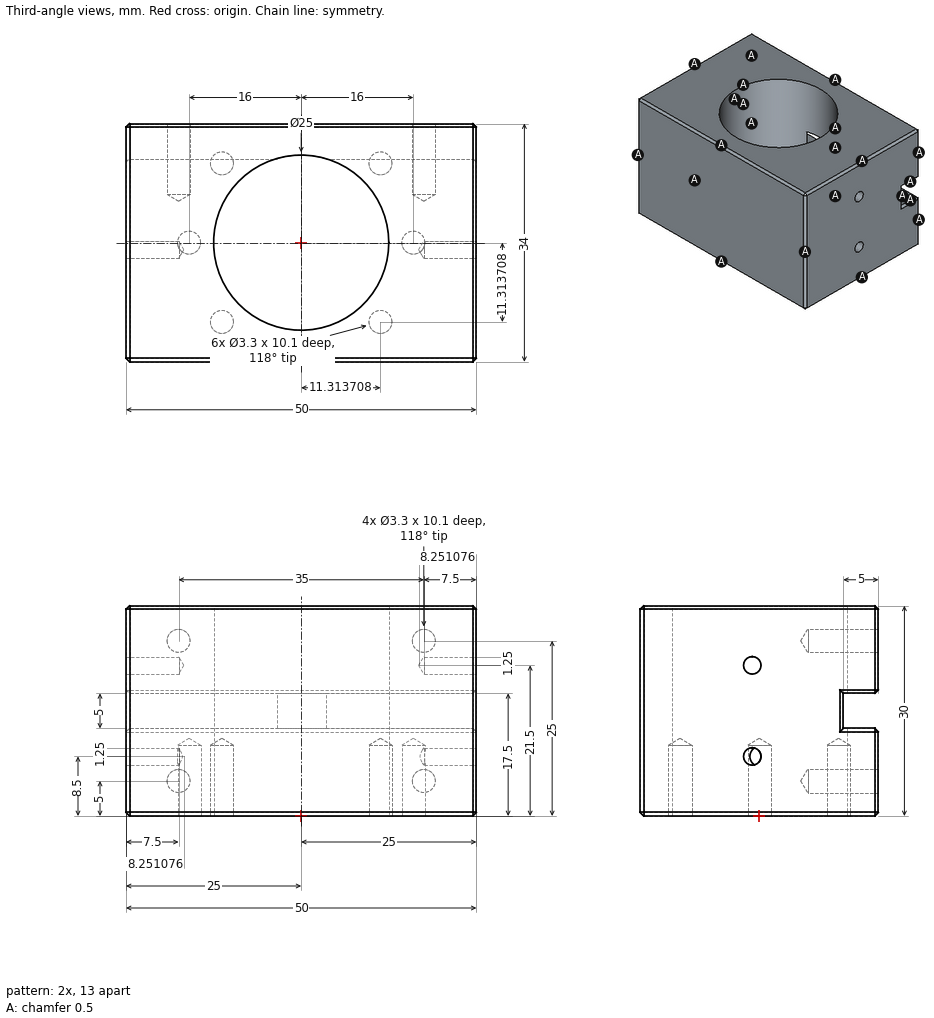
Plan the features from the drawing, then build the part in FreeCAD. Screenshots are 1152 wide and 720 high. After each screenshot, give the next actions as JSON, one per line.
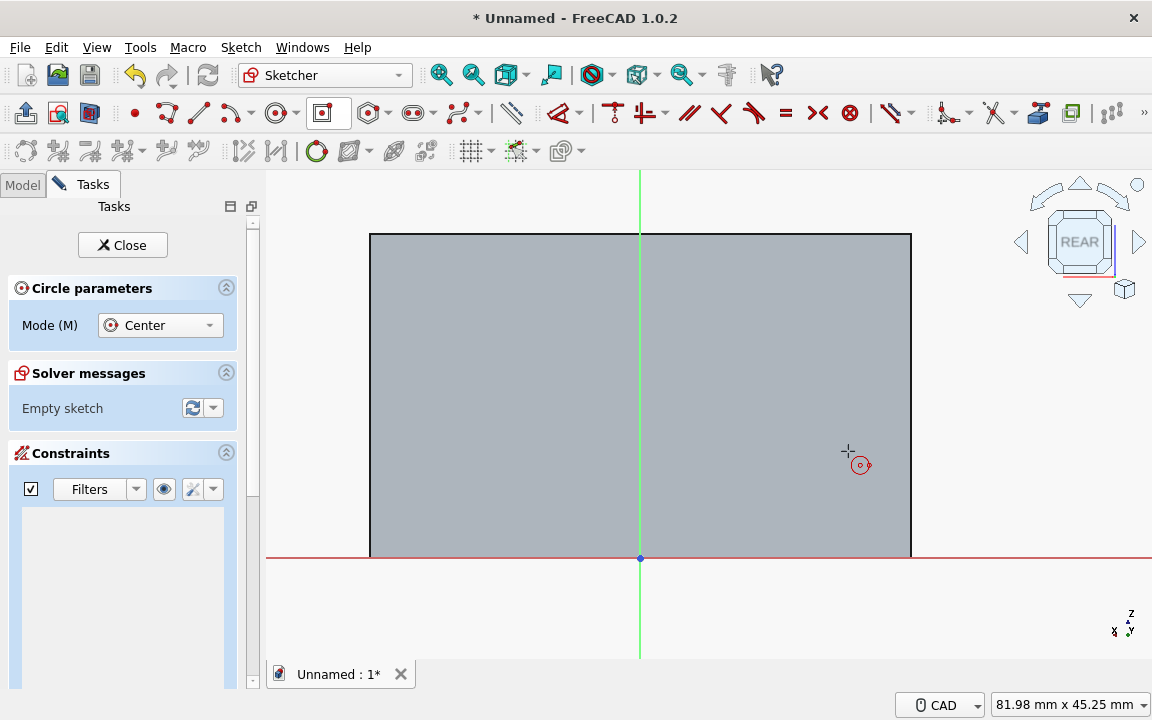
{"action": "scroll", "coordinate": [451, 288], "scroll_direction": "up", "scroll_amount": 2}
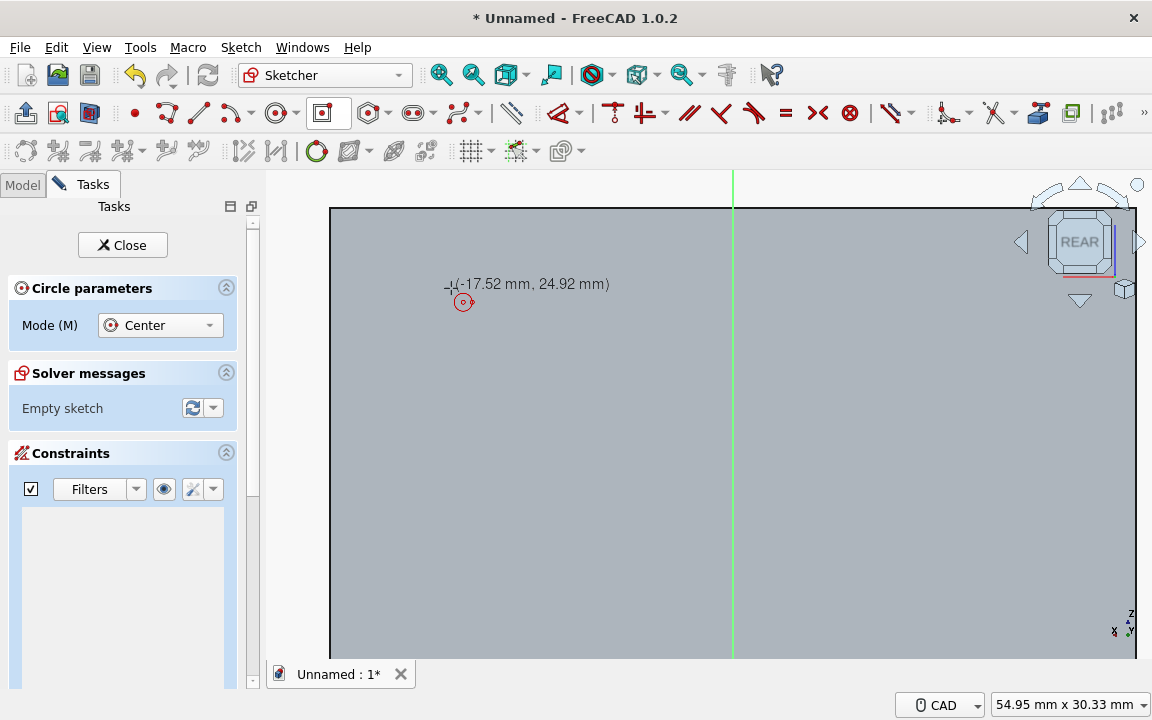
{"action": "left_click", "coordinate": [451, 288]}
{"action": "mouse_move", "coordinate": [470, 269]}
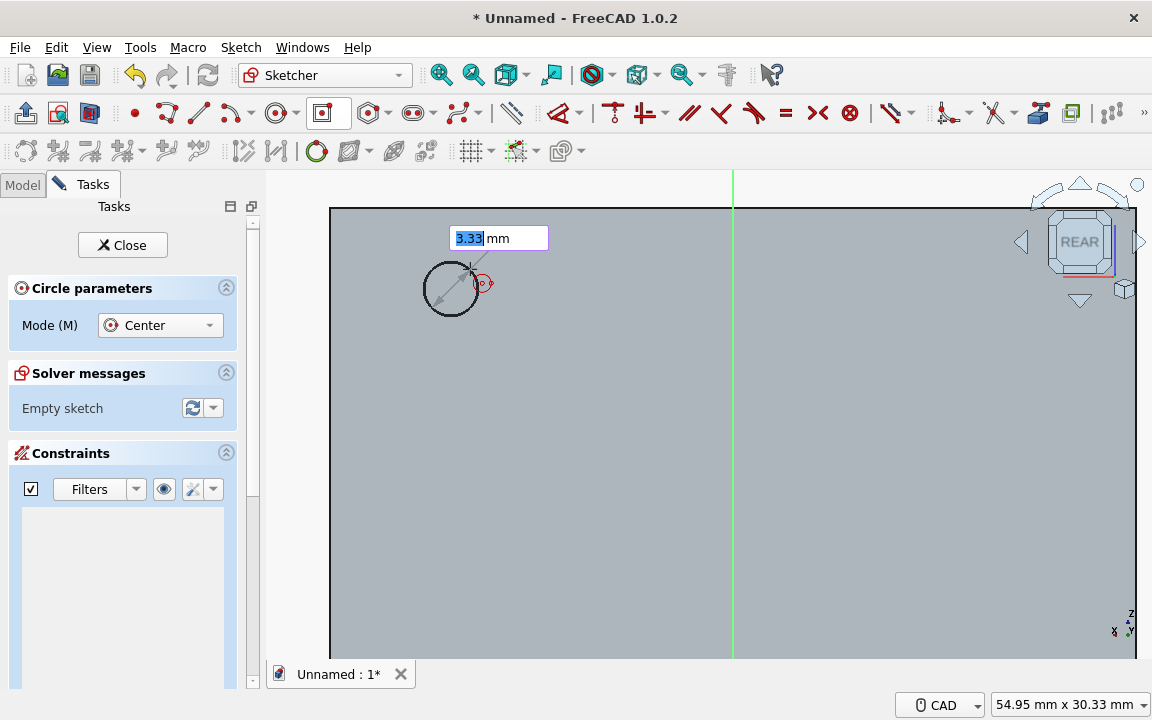
{"action": "type", "text": "3.3"}
{"action": "key", "text": "Return"}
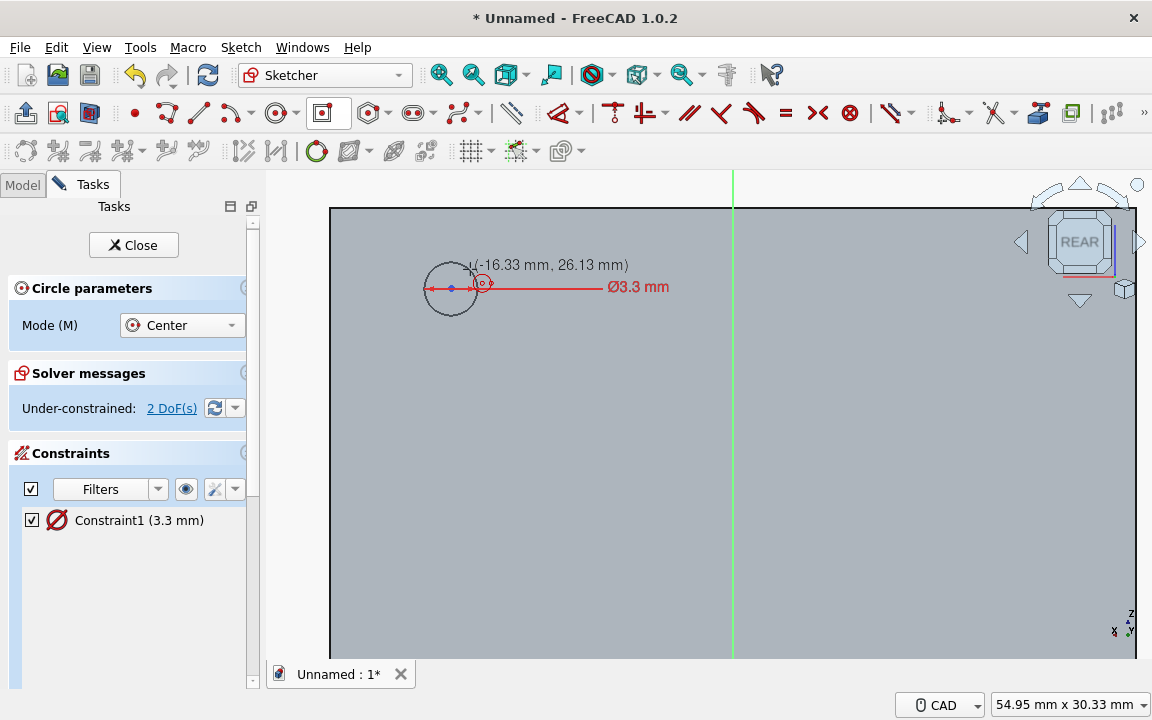
{"action": "scroll", "coordinate": [452, 289], "scroll_direction": "down", "scroll_amount": 2}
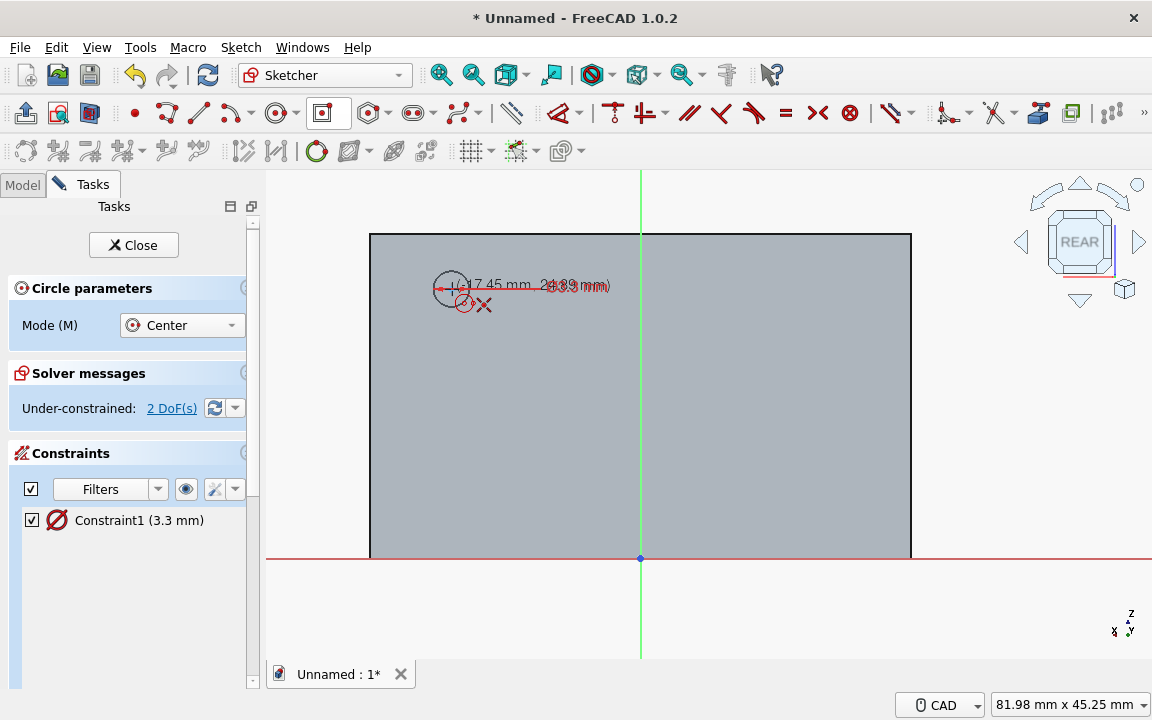
{"action": "scroll", "coordinate": [830, 289], "scroll_direction": "up", "scroll_amount": 2}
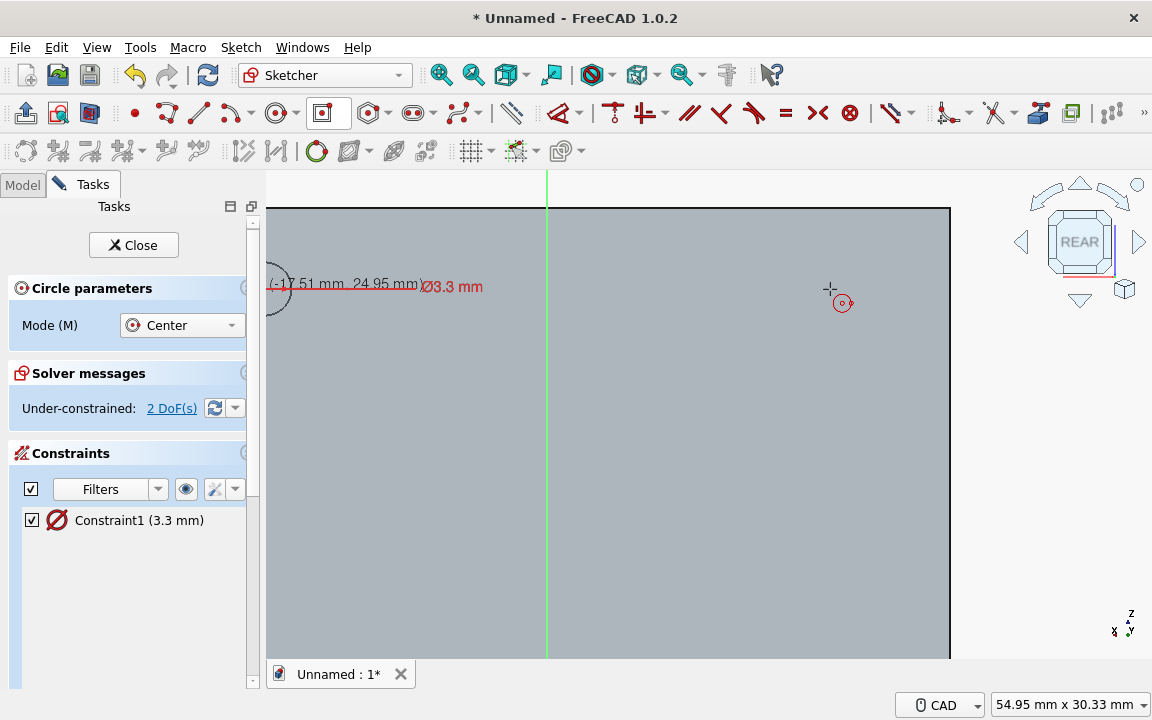
{"action": "left_click", "coordinate": [829, 288]}
{"action": "mouse_move", "coordinate": [848, 269]}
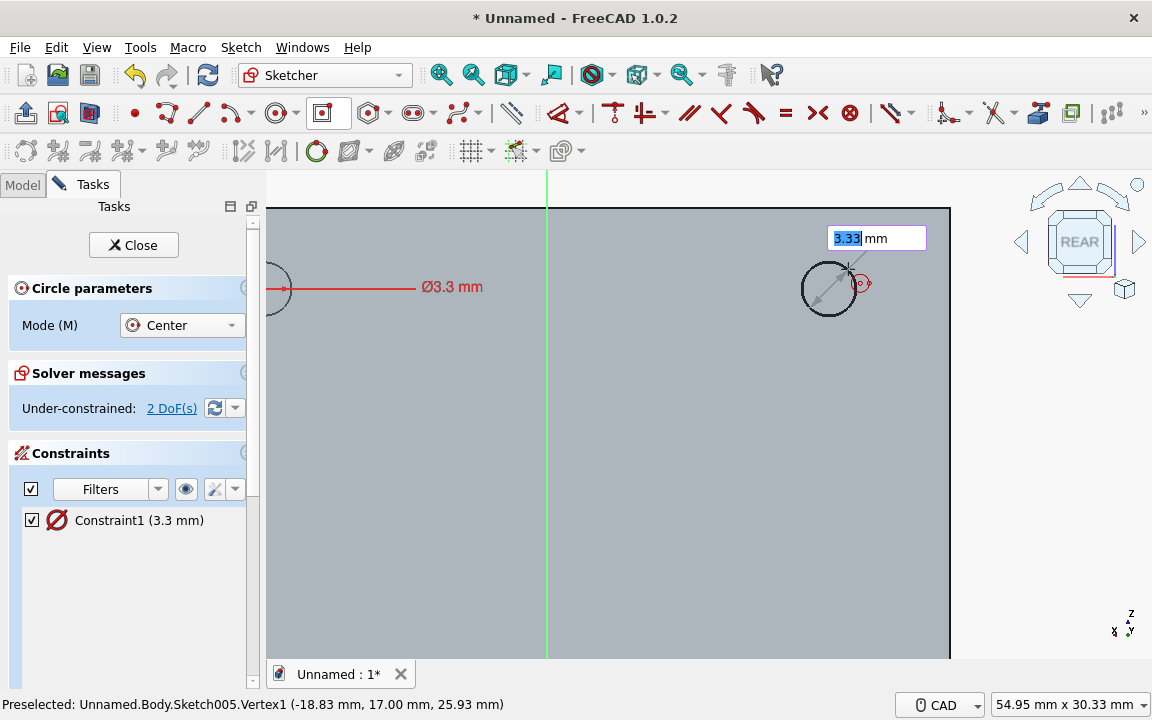
{"action": "type", "text": "3.3"}
{"action": "key", "text": "Return"}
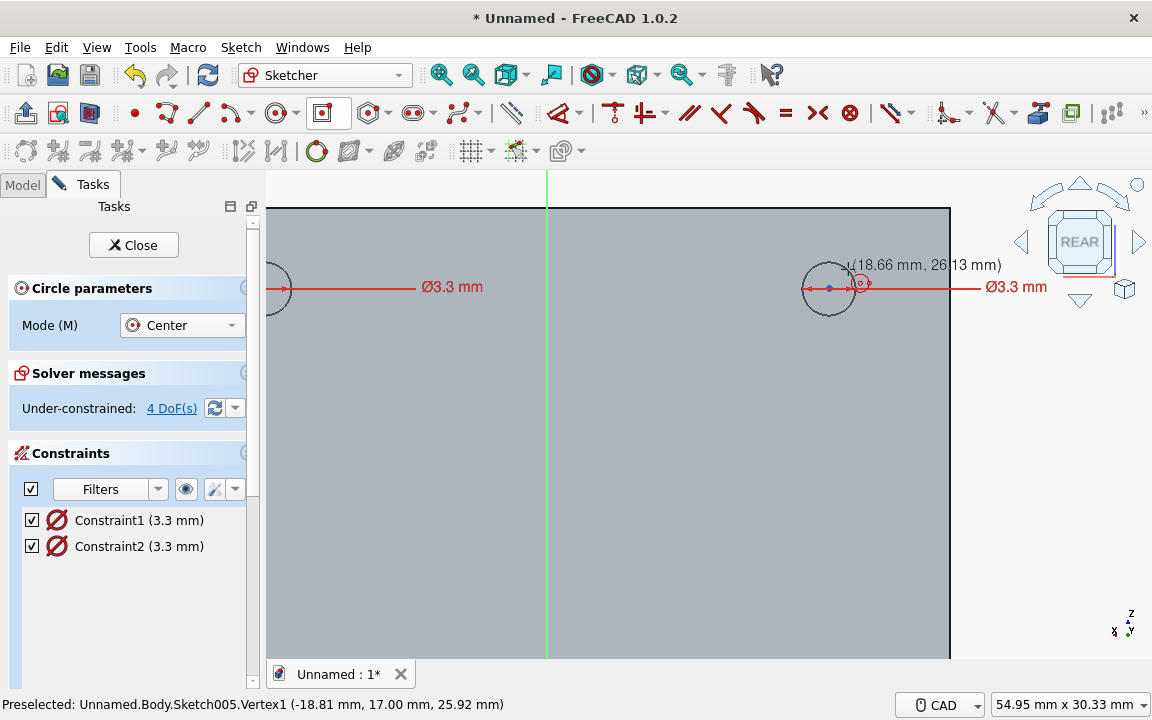
{"action": "left_click", "coordinate": [829, 611]}
{"action": "mouse_move", "coordinate": [848, 592]}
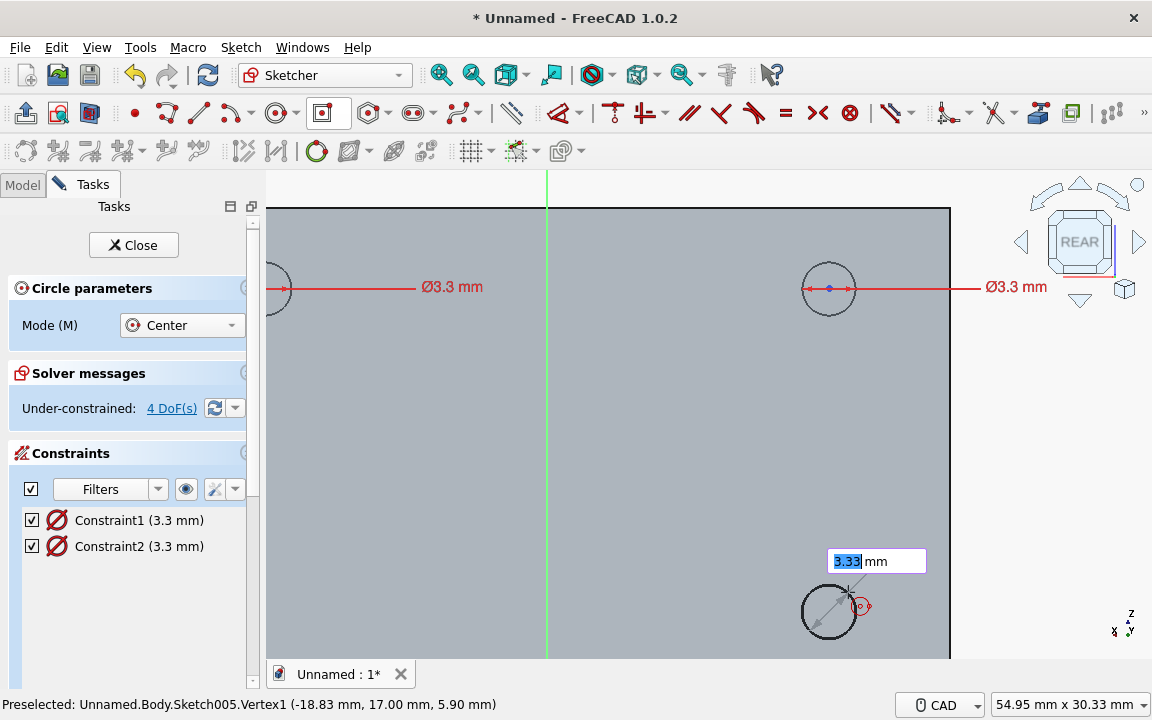
{"action": "type", "text": "3.3"}
{"action": "key", "text": "Return"}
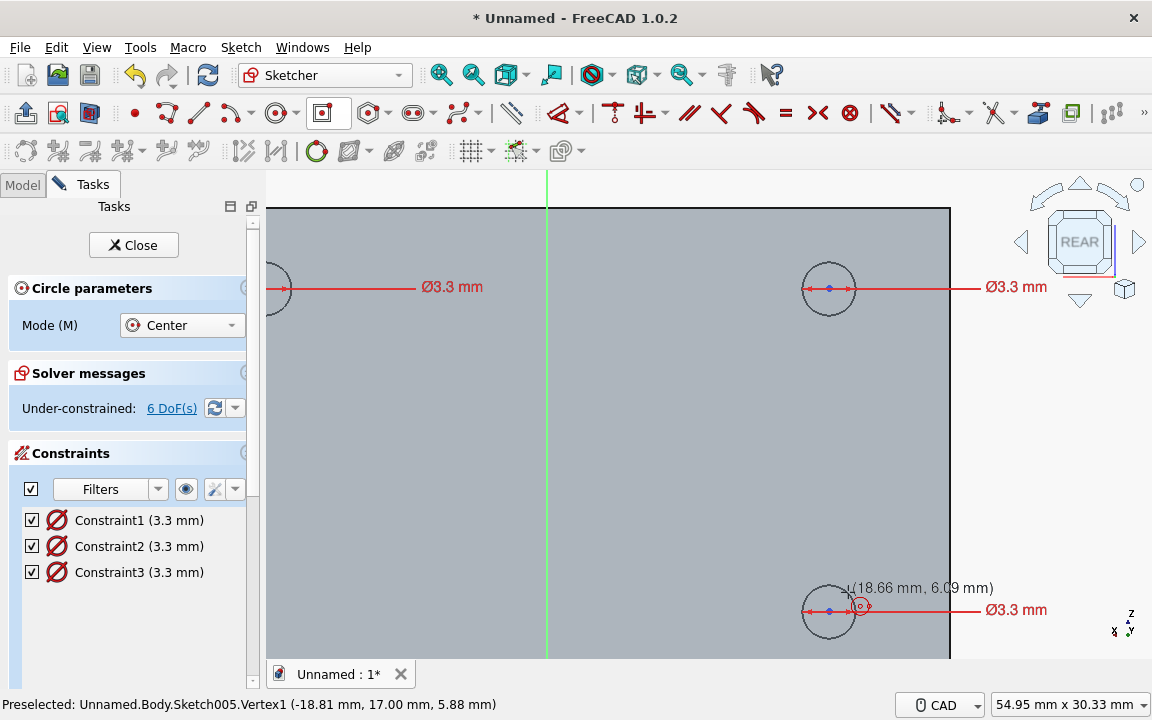
{"action": "scroll", "coordinate": [830, 289], "scroll_direction": "down", "scroll_amount": 2}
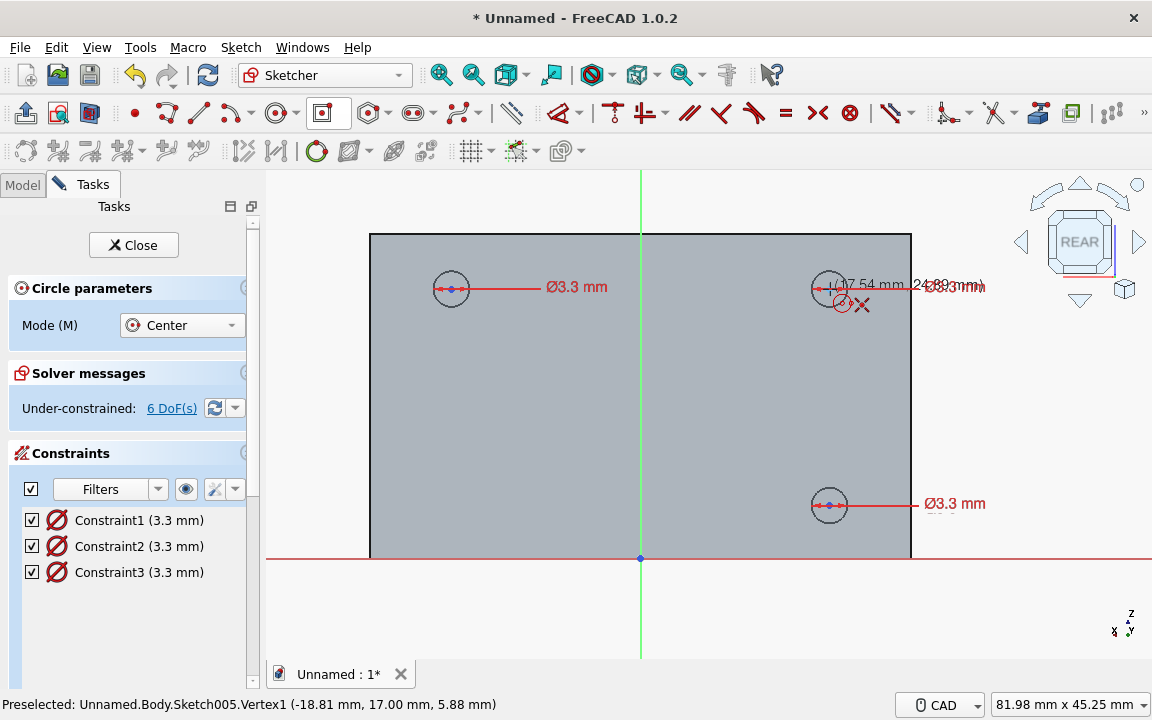
{"action": "scroll", "coordinate": [452, 505], "scroll_direction": "up", "scroll_amount": 2}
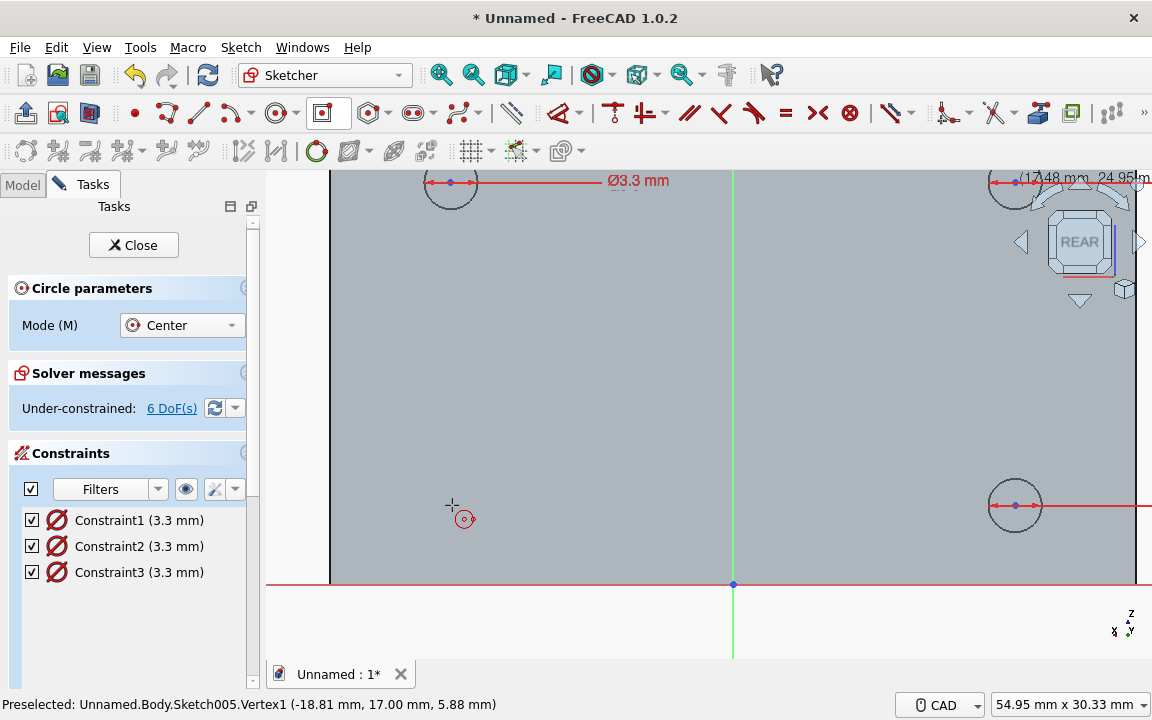
{"action": "left_click", "coordinate": [451, 504]}
{"action": "mouse_move", "coordinate": [470, 485]}